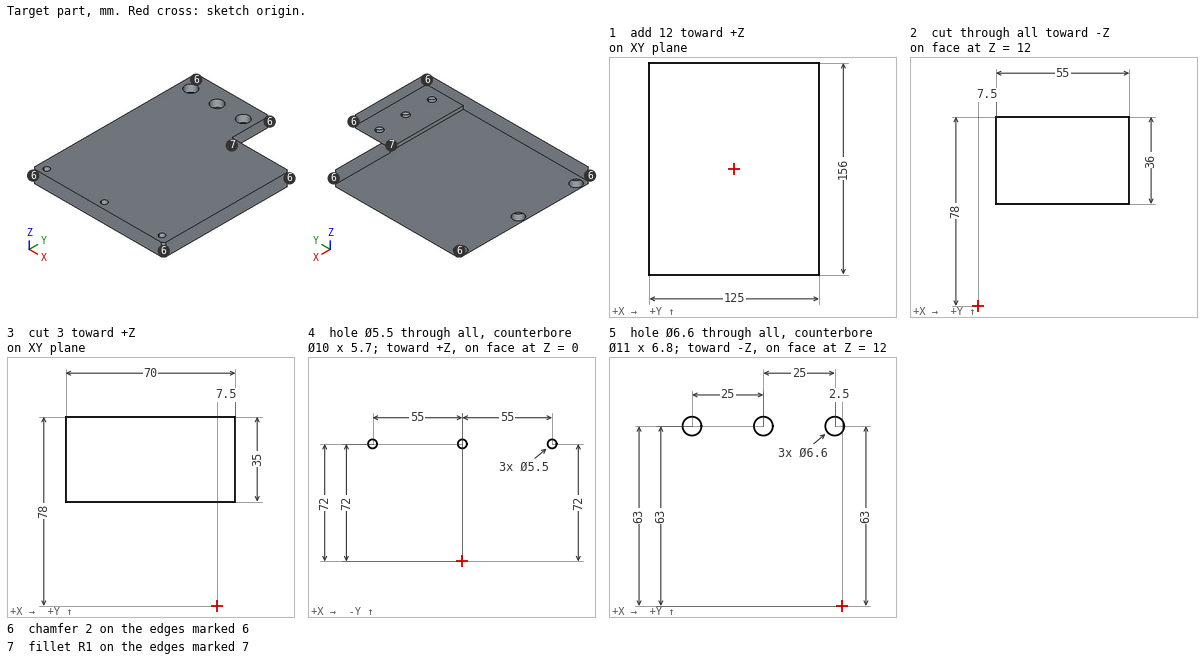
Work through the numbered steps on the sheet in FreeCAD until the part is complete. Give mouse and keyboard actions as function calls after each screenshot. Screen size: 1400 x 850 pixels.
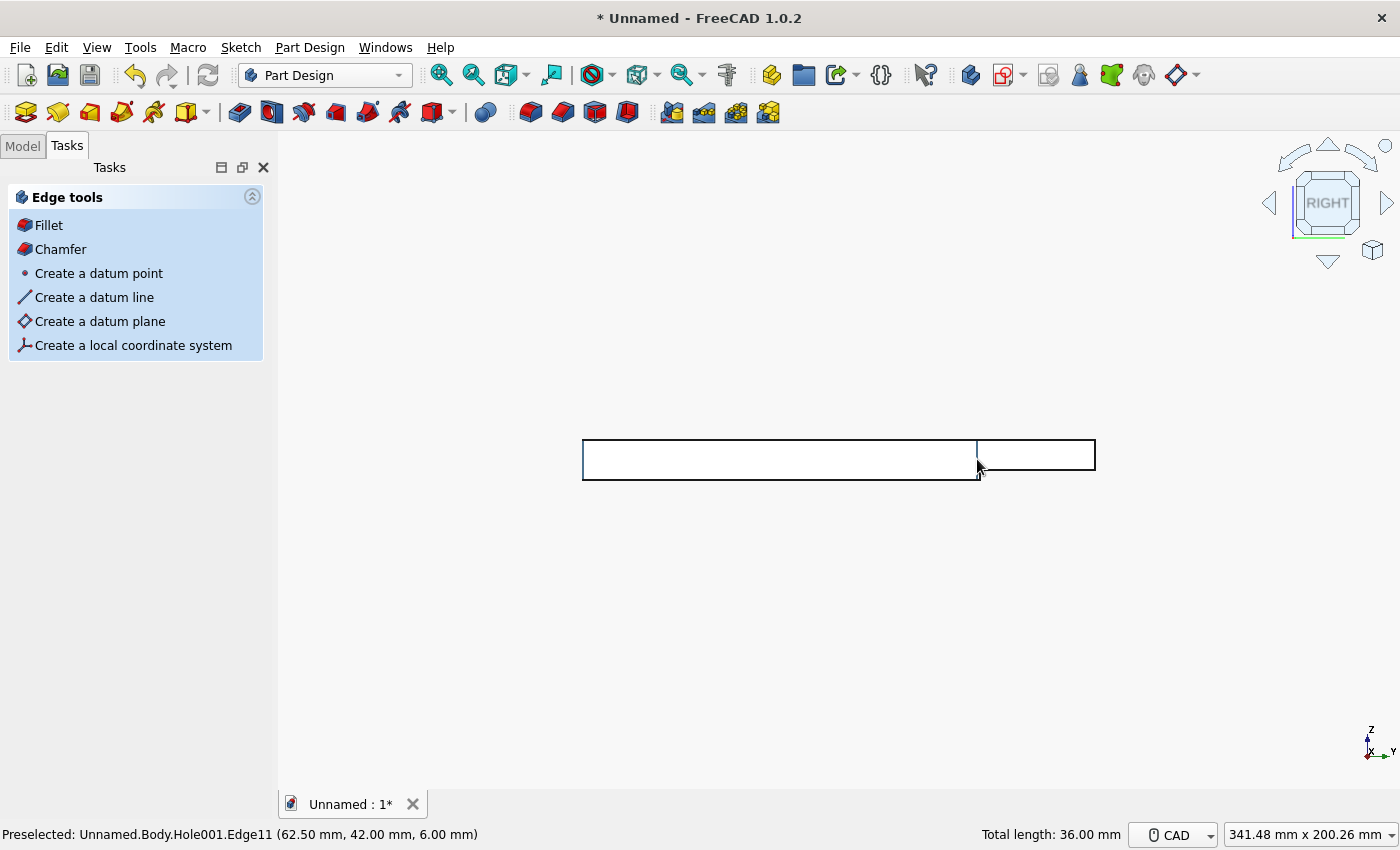
click(1095, 454, ctrl)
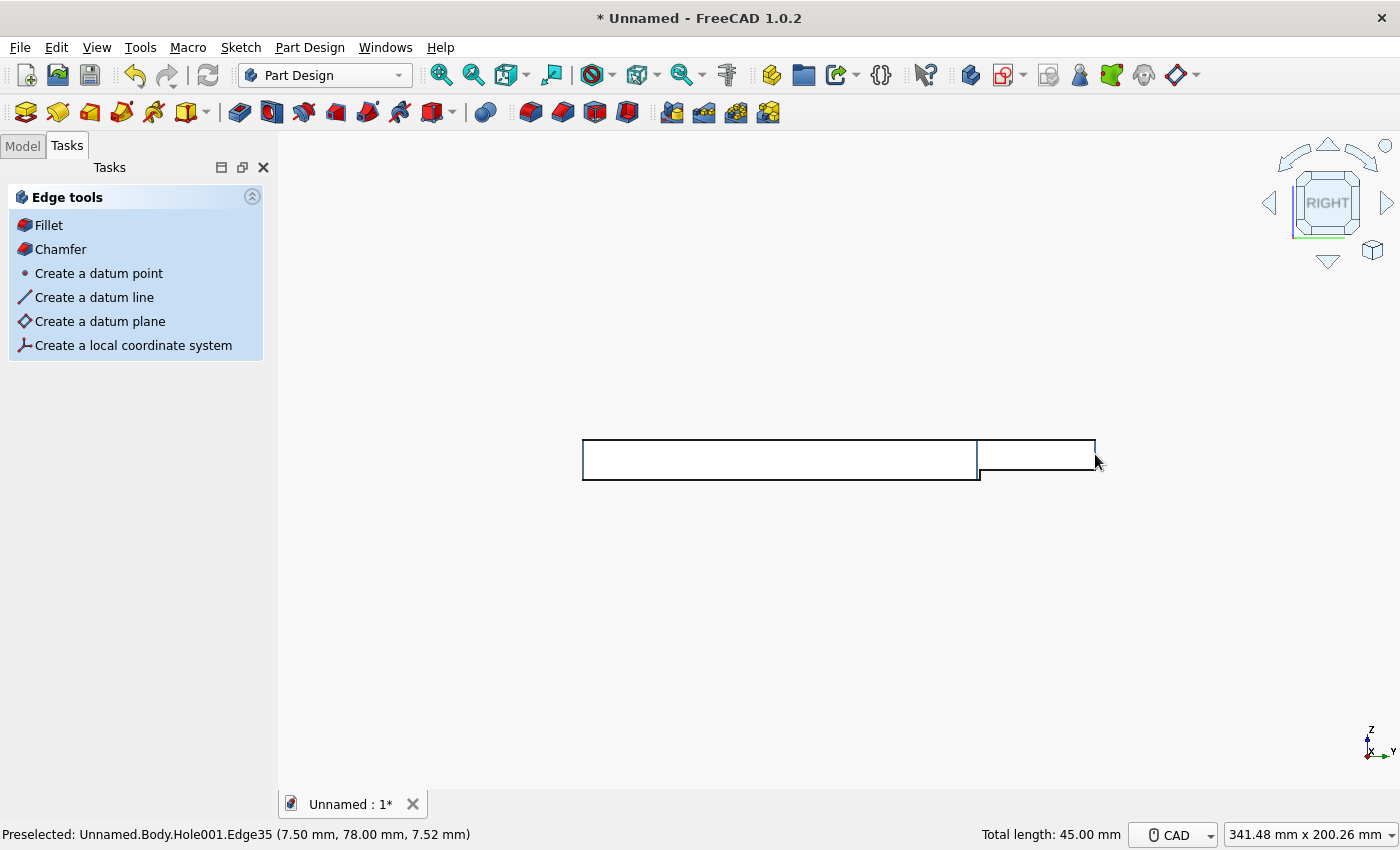
key(5)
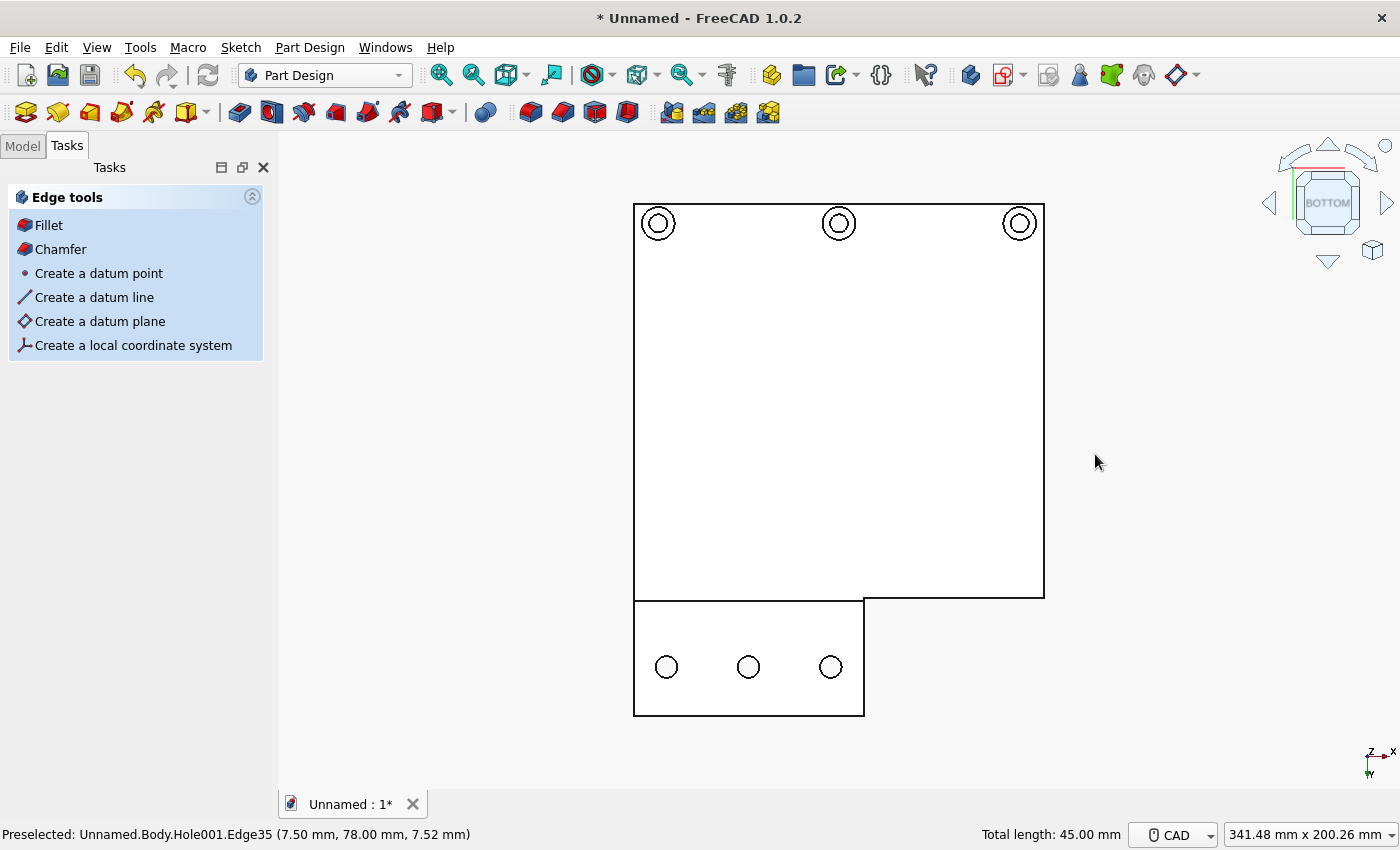
key(4)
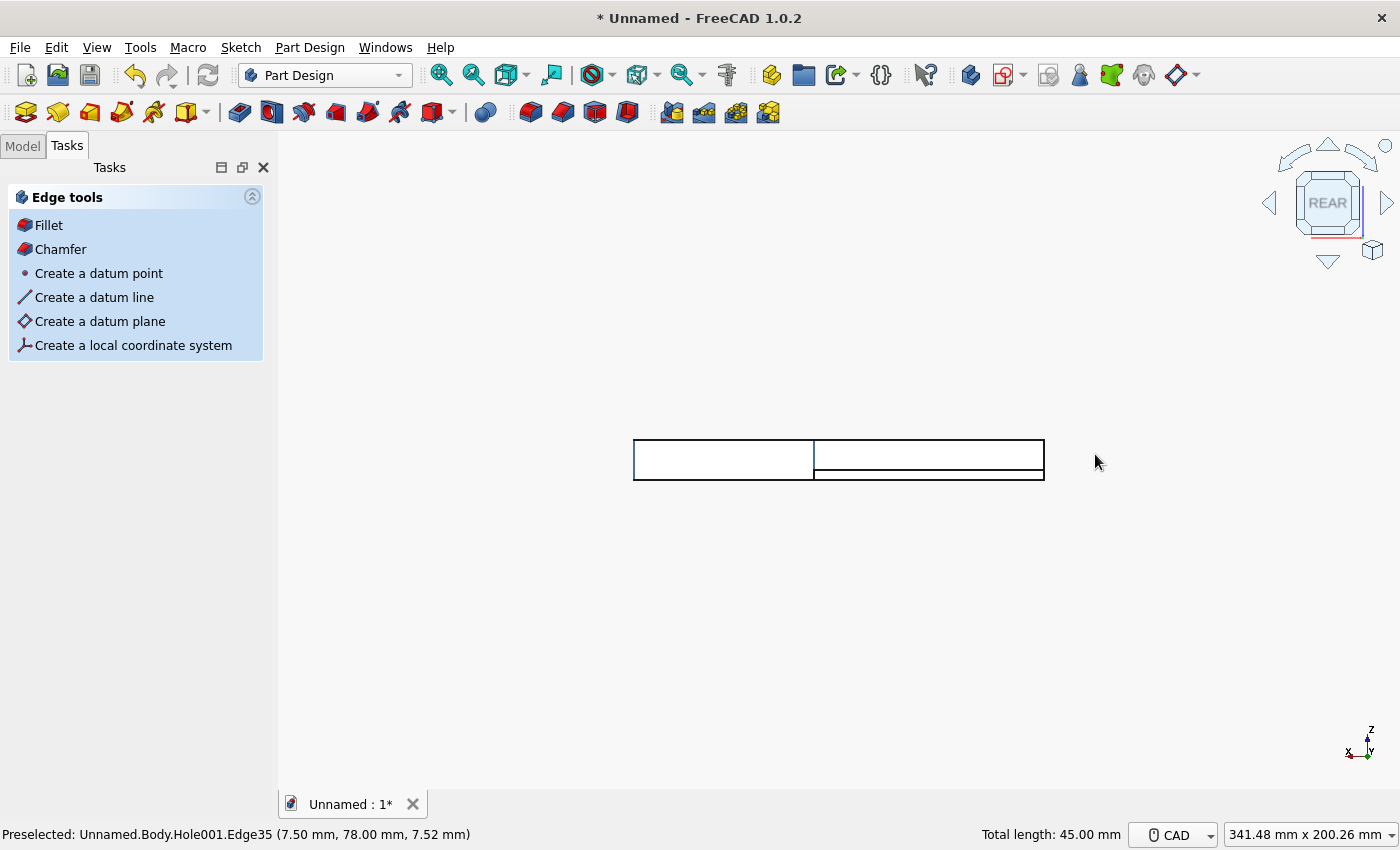
click(442, 76)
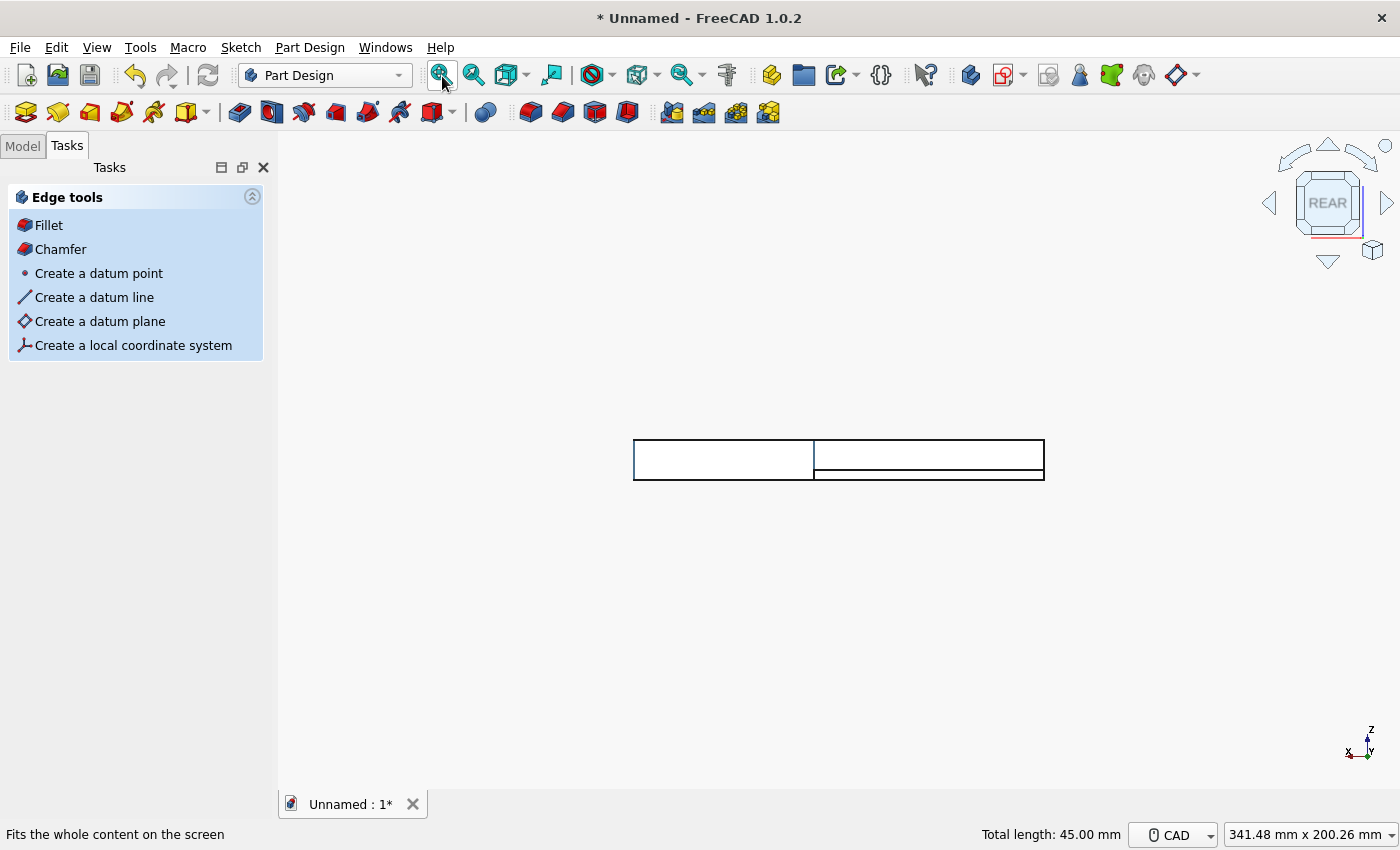
click(1044, 454, ctrl)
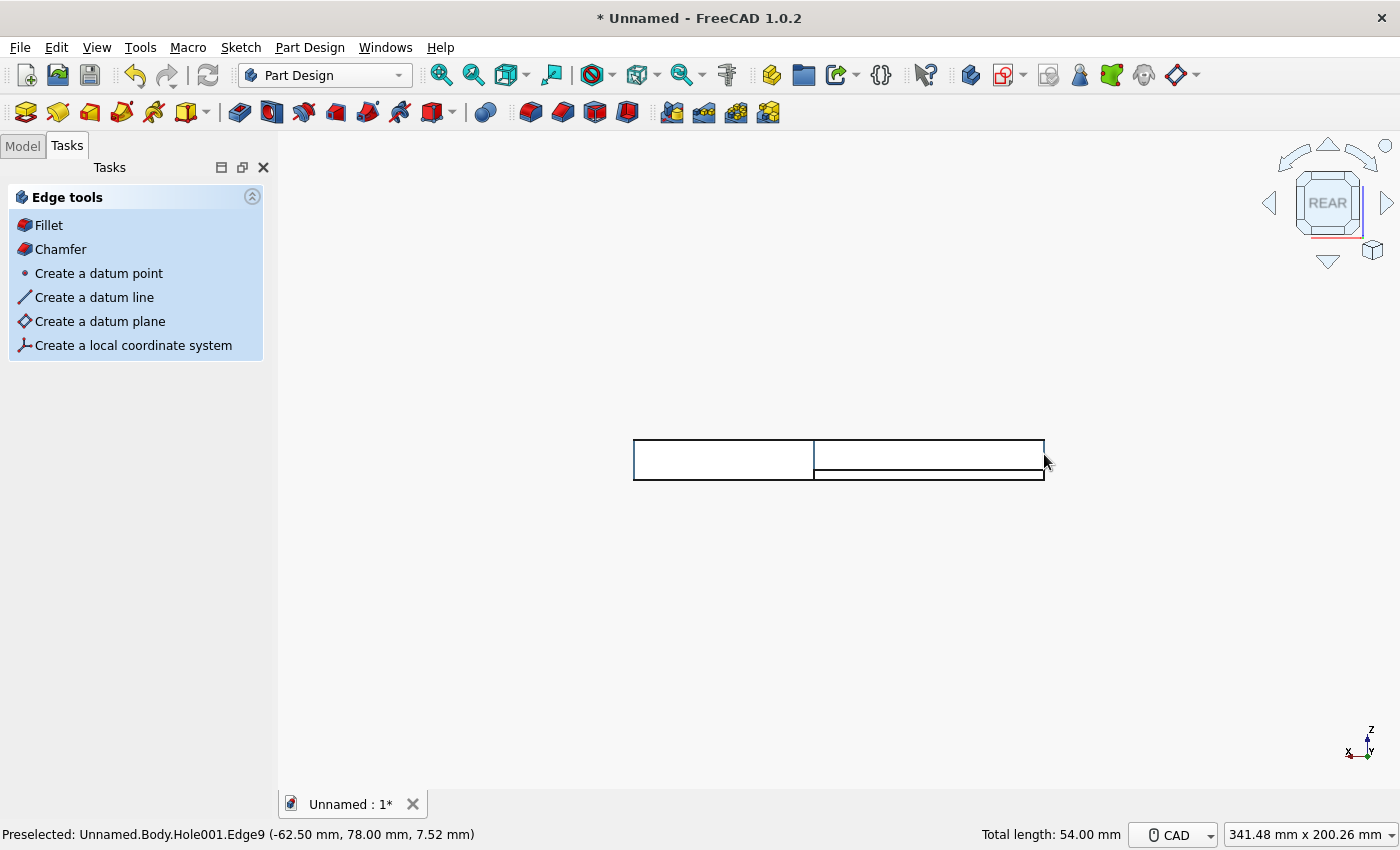
click(564, 112)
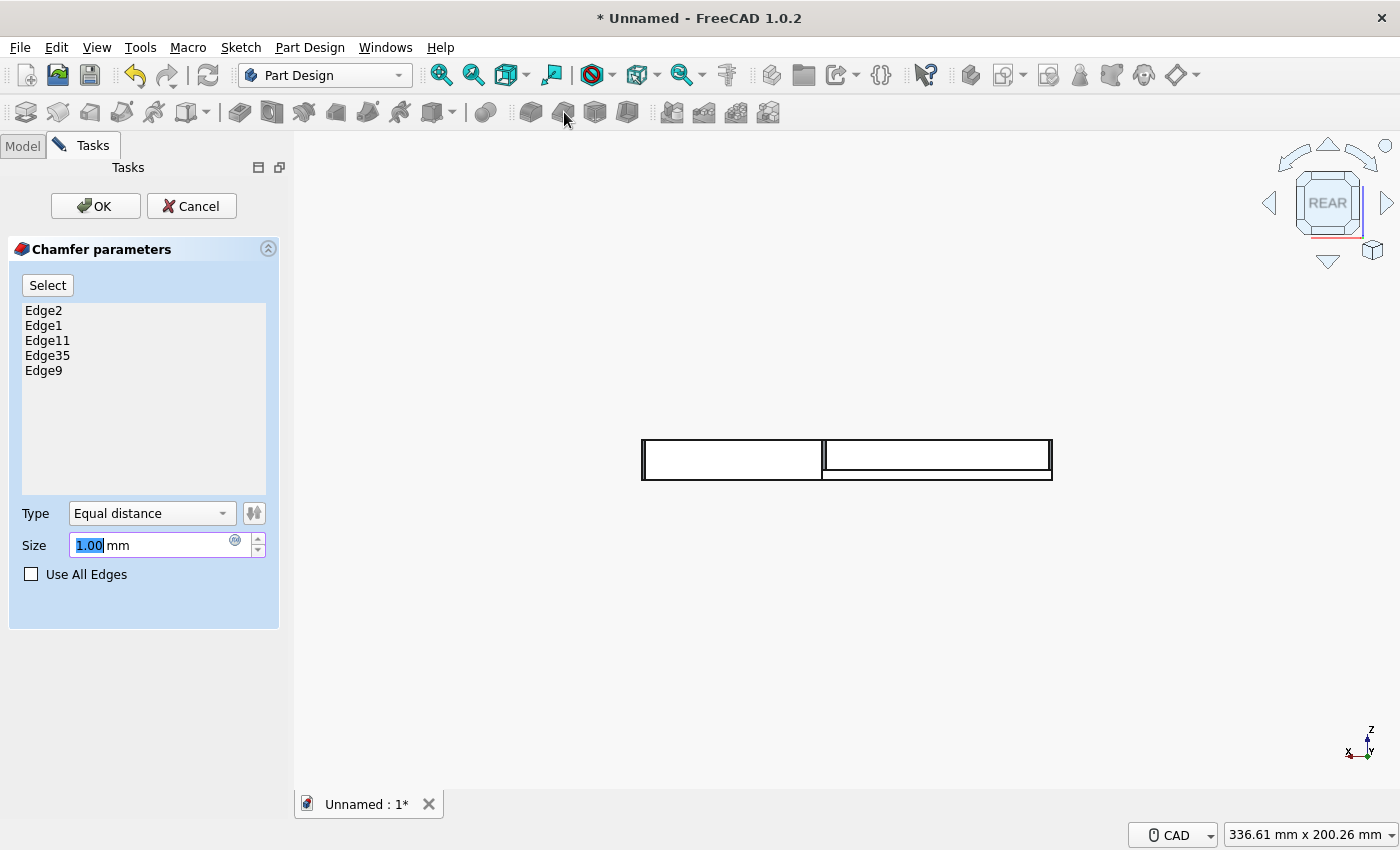
text(2)
key(Tab)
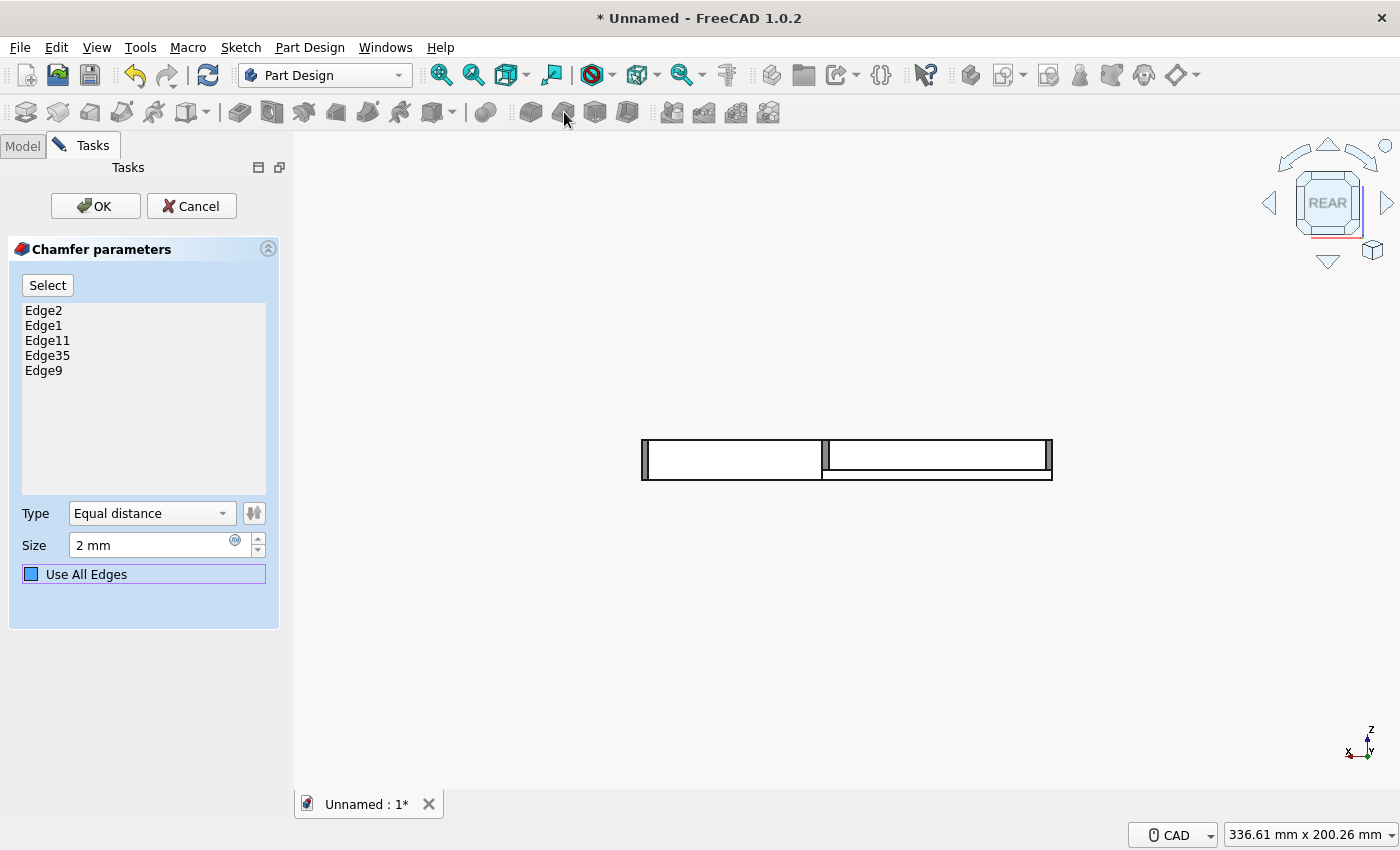
click(96, 206)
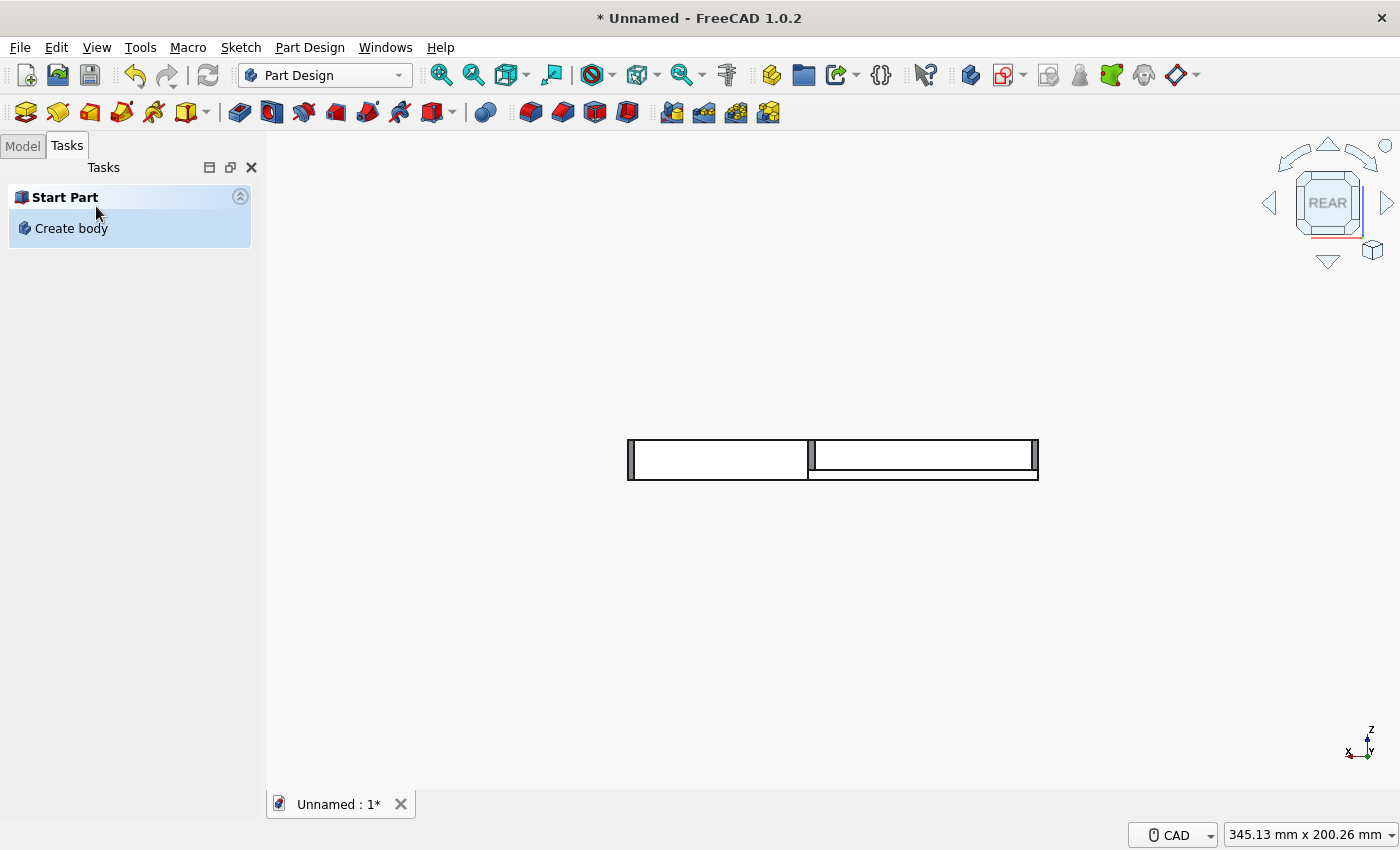
click(442, 76)